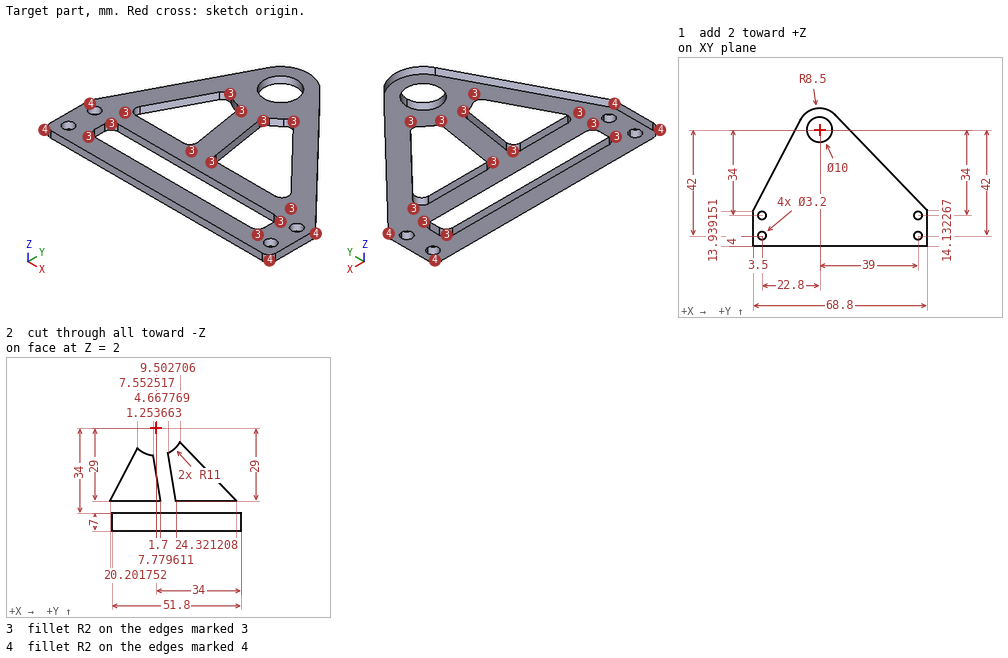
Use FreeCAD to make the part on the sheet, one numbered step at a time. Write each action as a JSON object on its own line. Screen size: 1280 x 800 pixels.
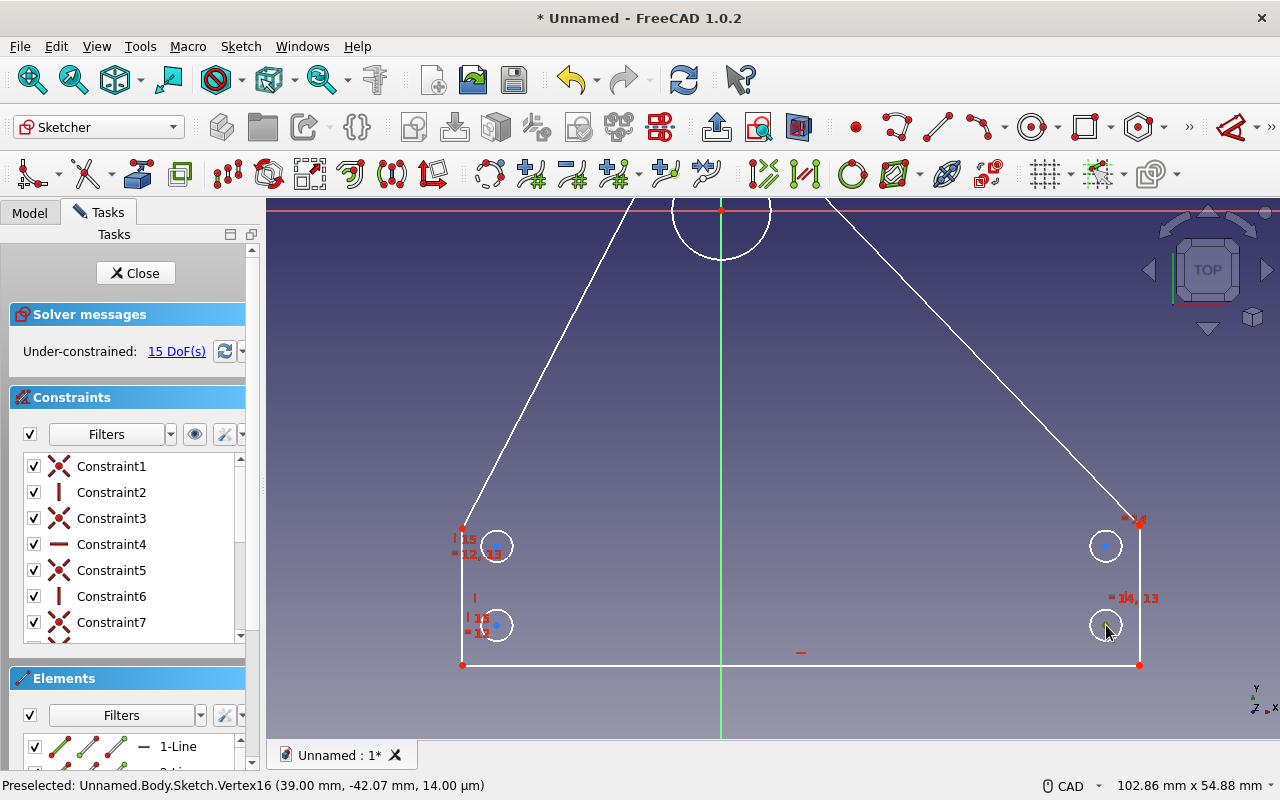
{"action": "left_click", "coordinate": [1106, 546]}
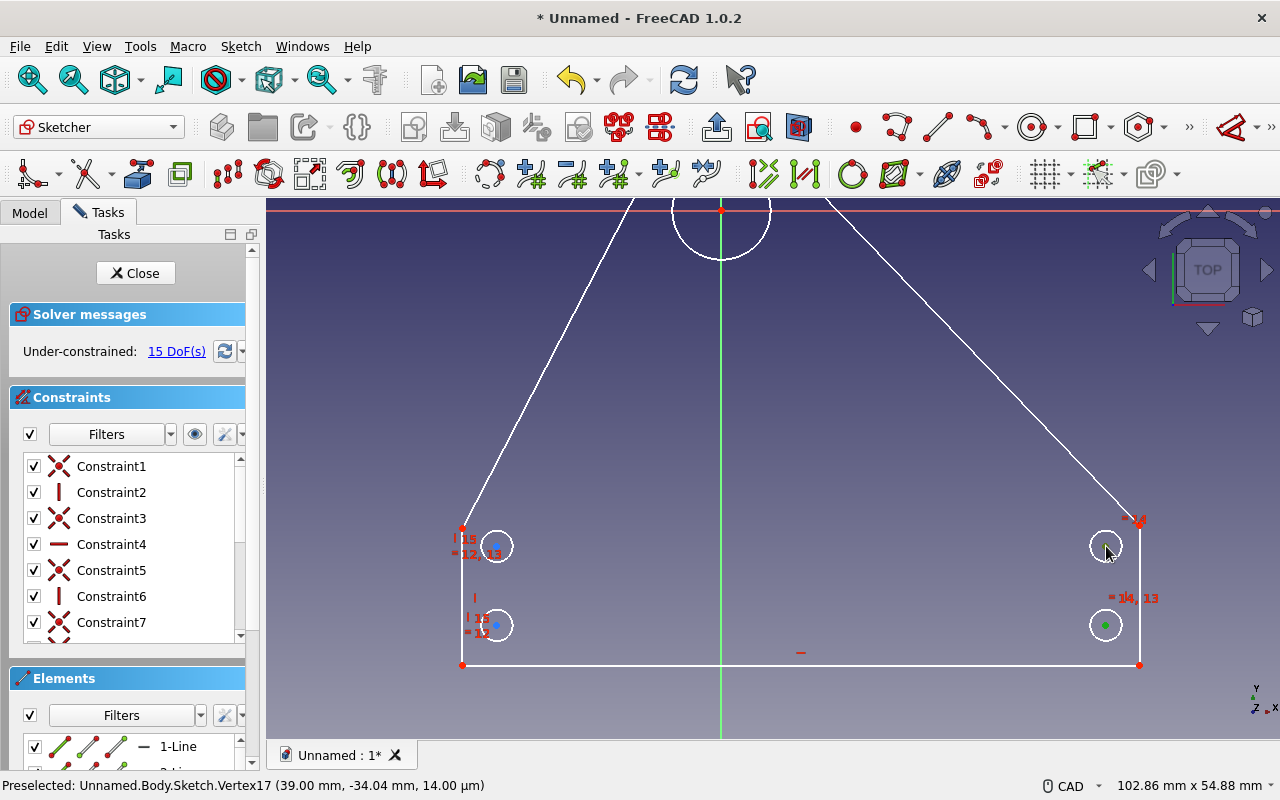
{"action": "key", "text": "v"}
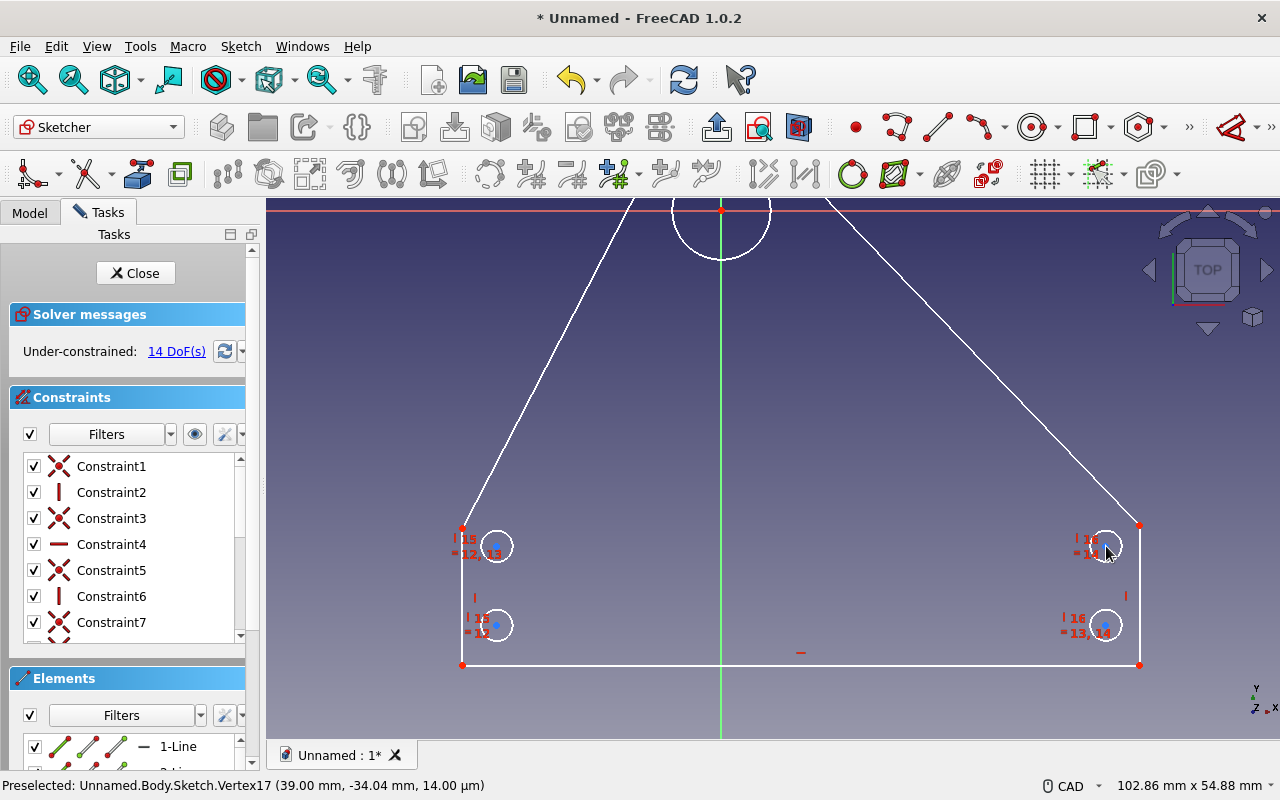
{"action": "left_click", "coordinate": [1230, 128]}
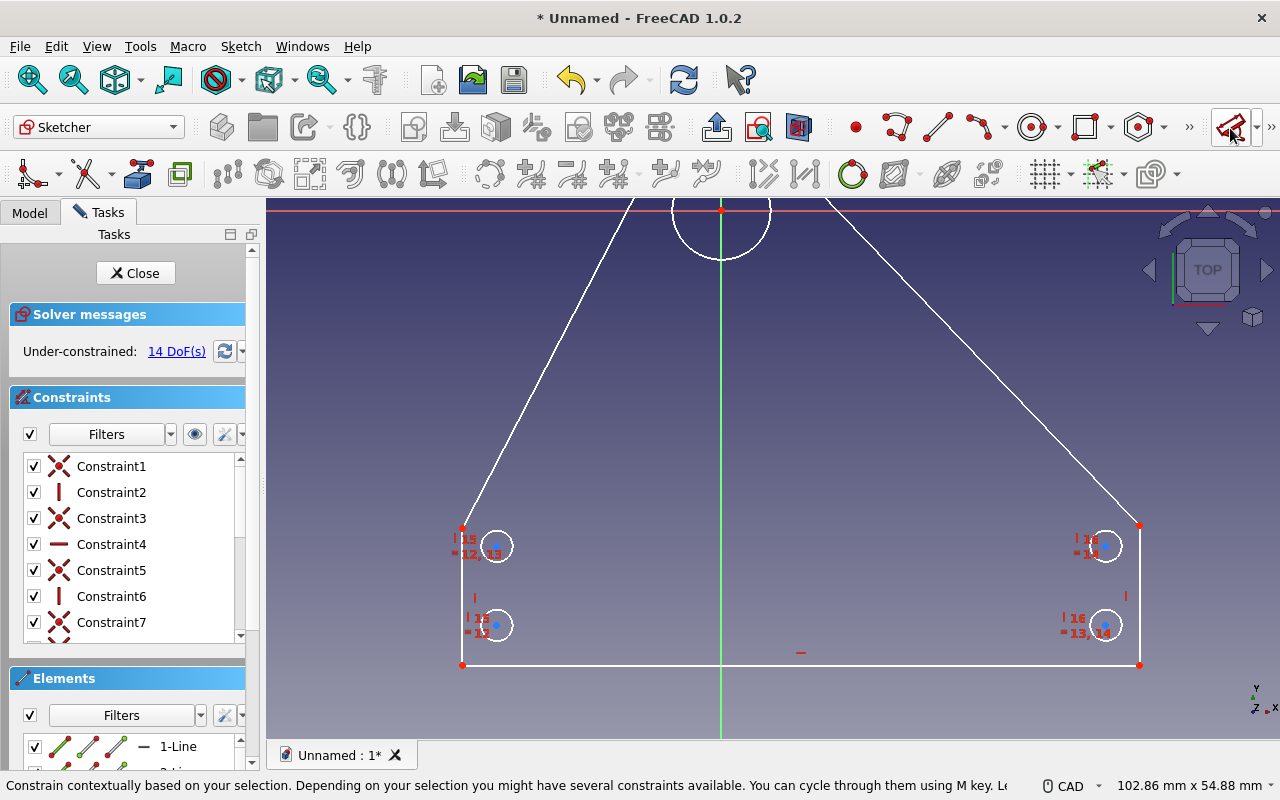
{"action": "scroll", "coordinate": [508, 616], "scroll_direction": "down", "scroll_amount": 2}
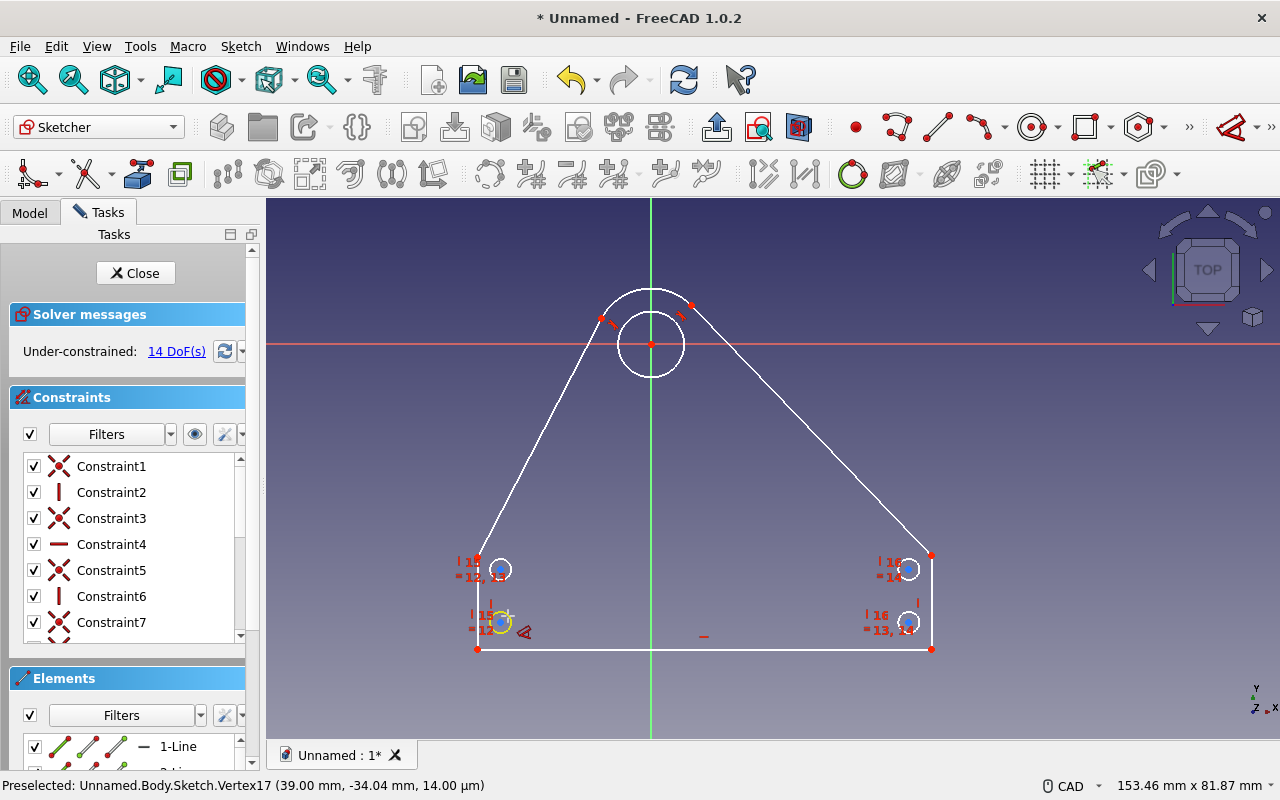
{"action": "left_click", "coordinate": [664, 290]}
{"action": "left_click", "coordinate": [671, 259]}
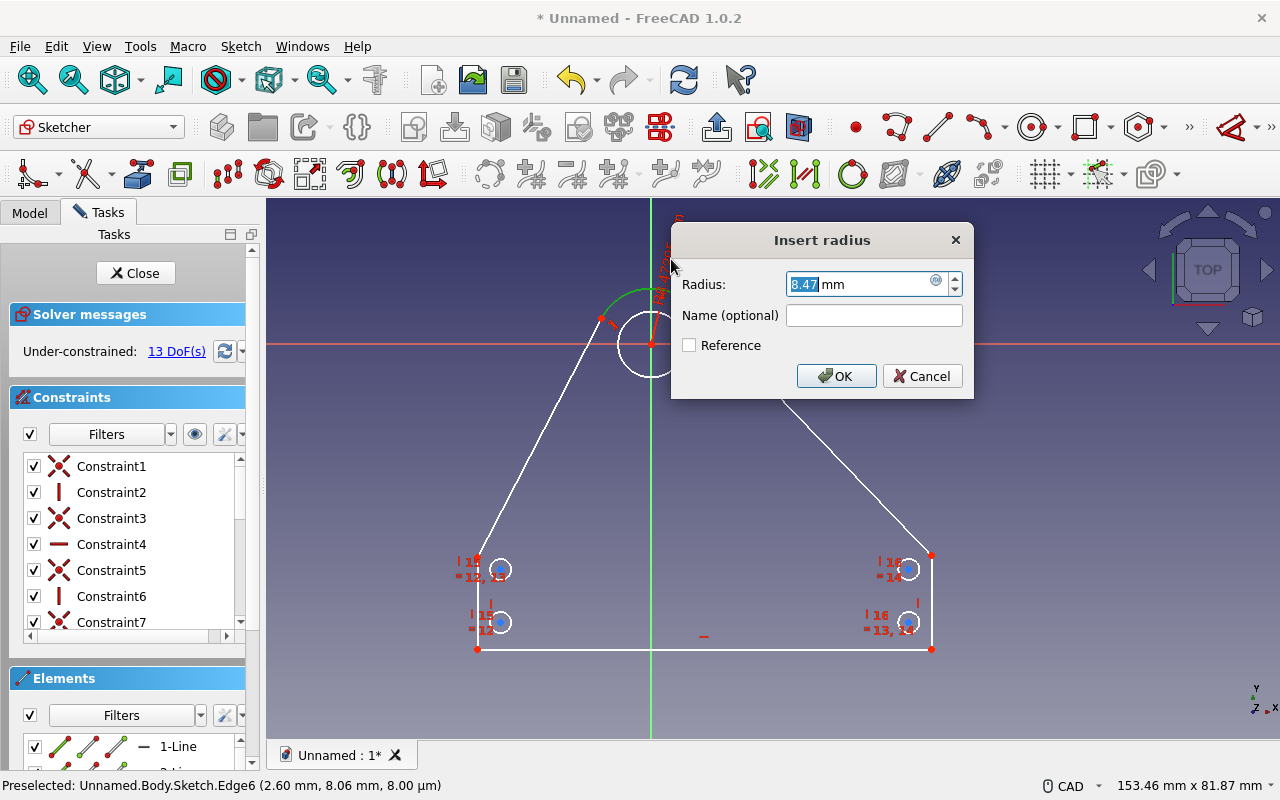
{"action": "type", "text": "8.5"}
{"action": "key", "text": "Return"}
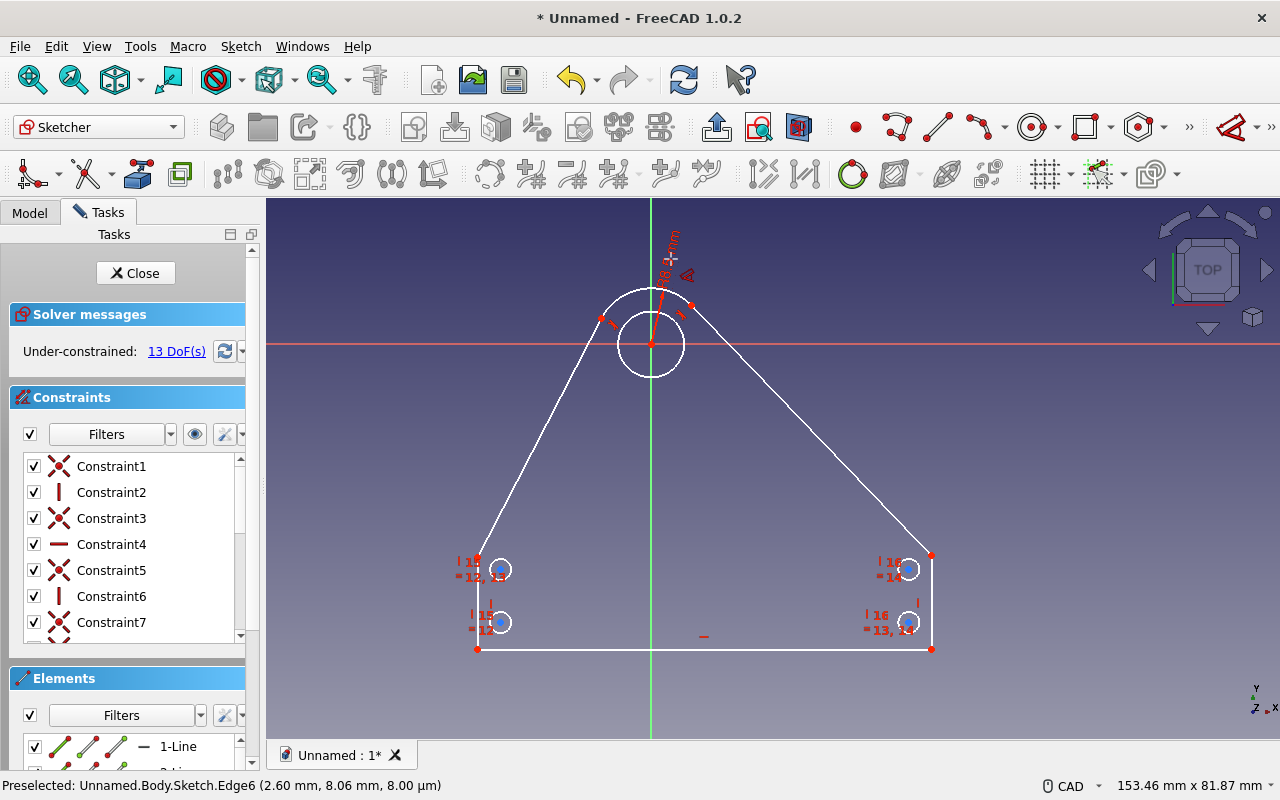
{"action": "scroll", "coordinate": [508, 615], "scroll_direction": "up", "scroll_amount": 4}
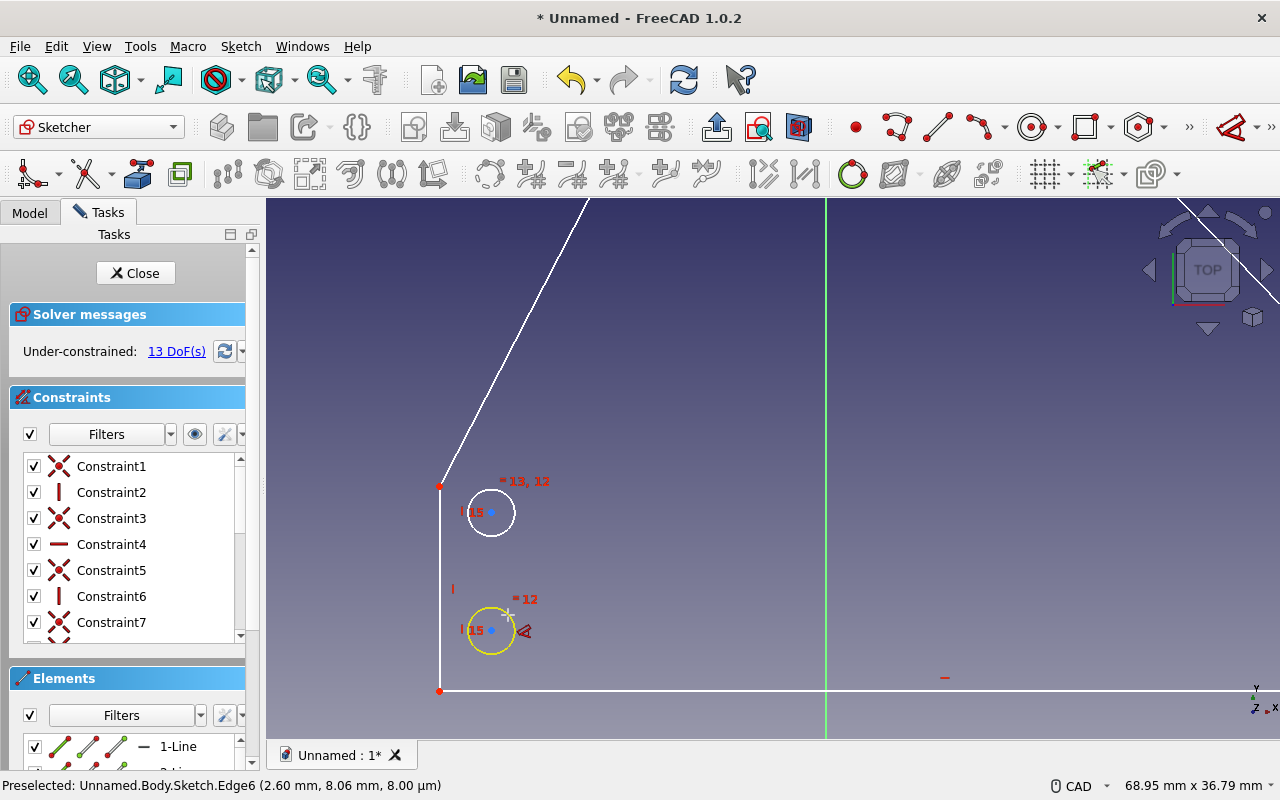
{"action": "left_click", "coordinate": [508, 614]}
{"action": "left_click", "coordinate": [530, 591]}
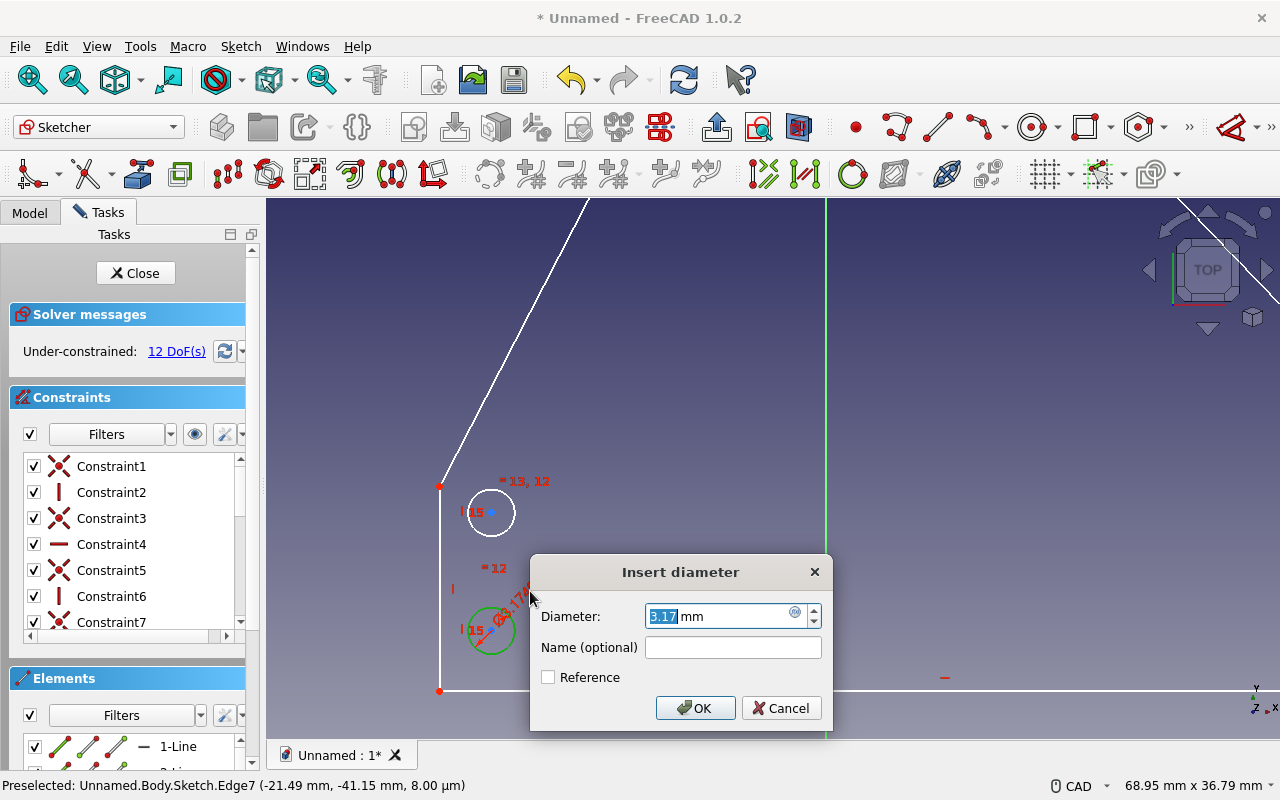
{"action": "type", "text": "3.2"}
{"action": "key", "text": "Return"}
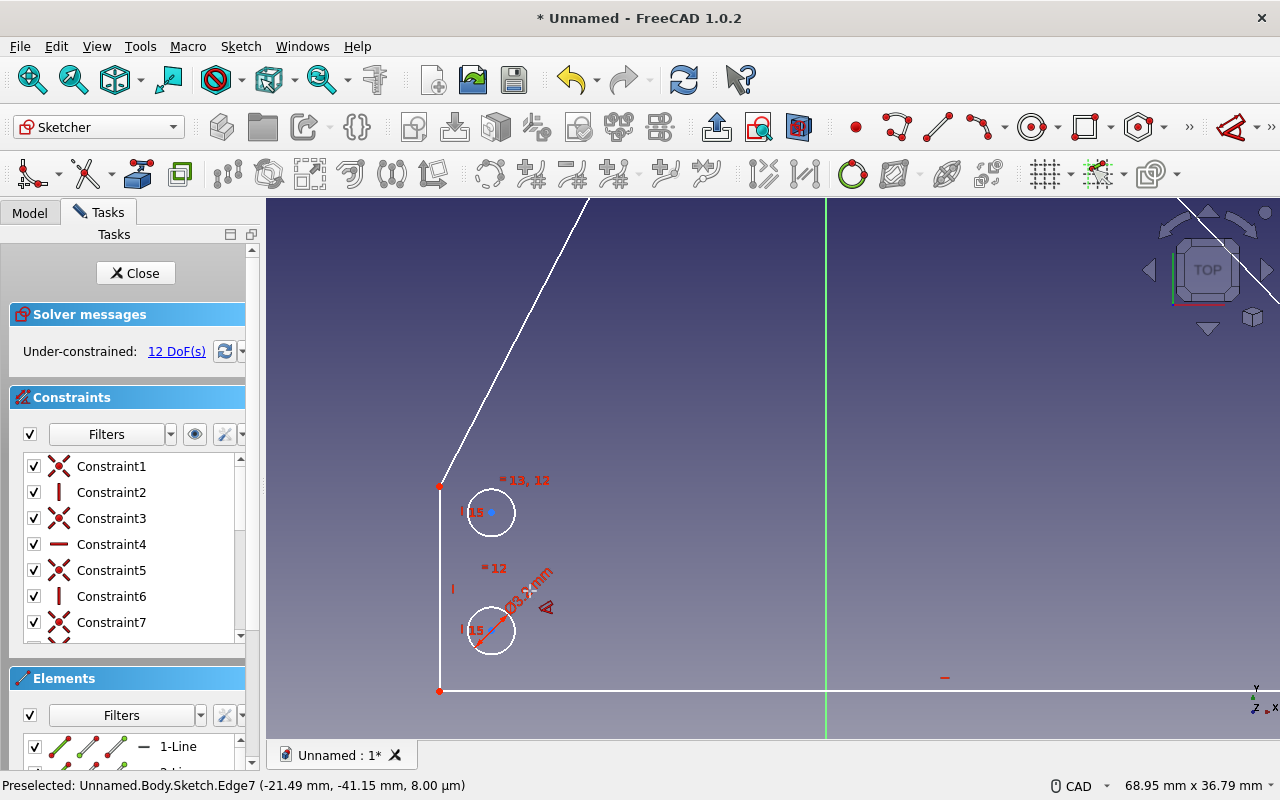
{"action": "scroll", "coordinate": [508, 615], "scroll_direction": "down", "scroll_amount": 4}